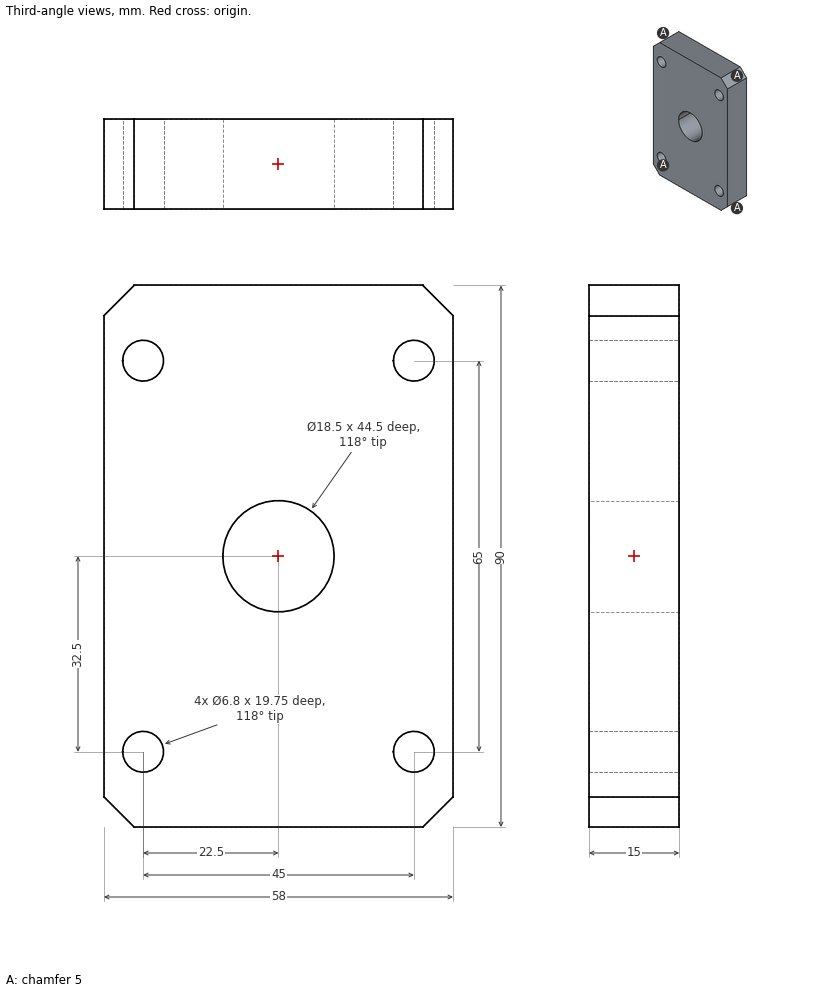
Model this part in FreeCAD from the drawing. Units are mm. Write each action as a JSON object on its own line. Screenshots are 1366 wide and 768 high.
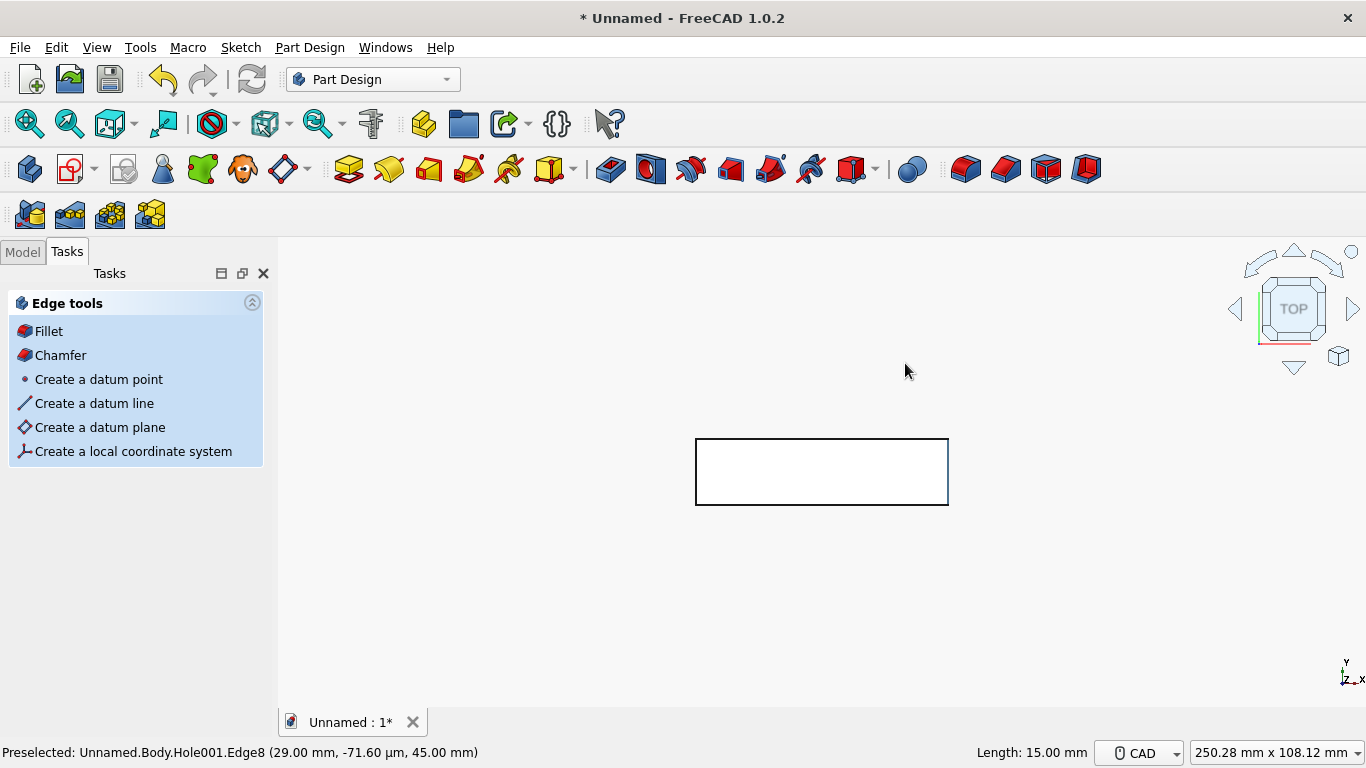
{"action": "left_click", "coordinate": [30, 124]}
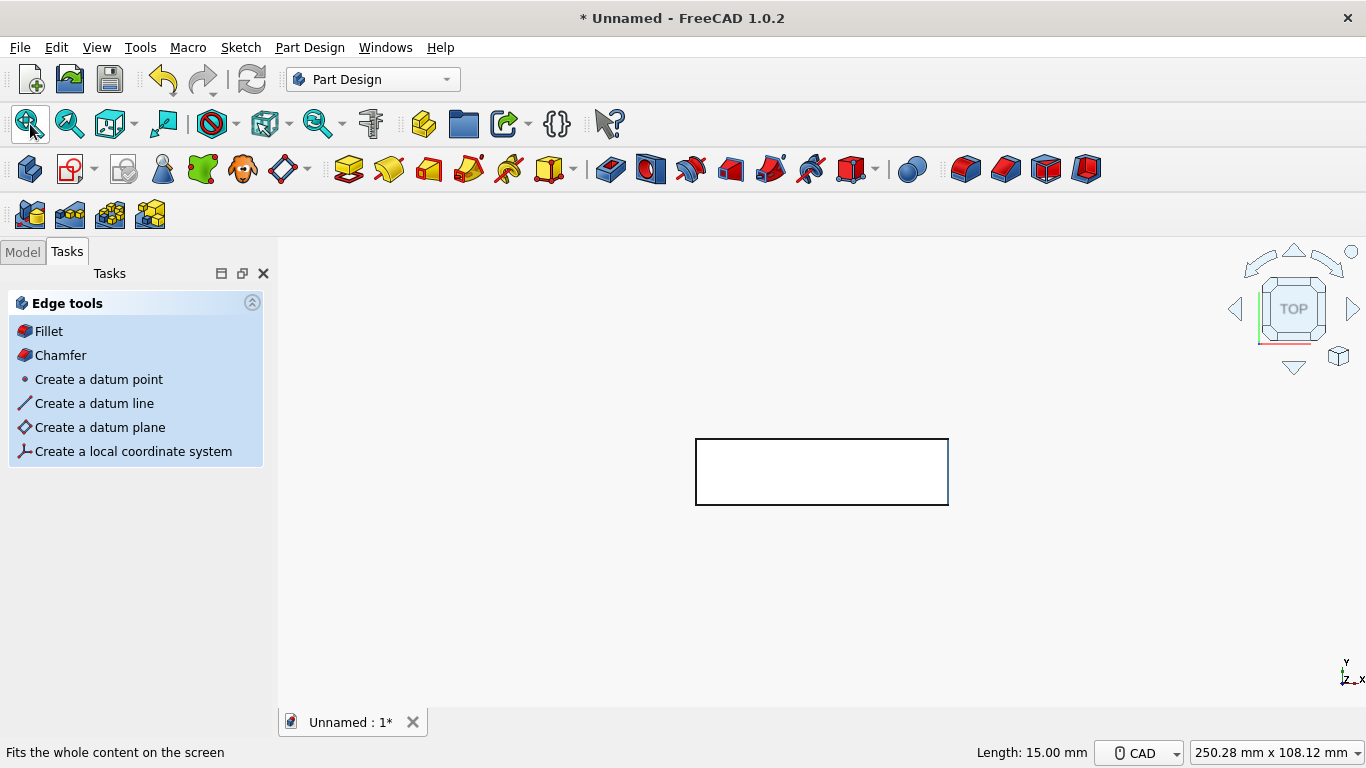
{"action": "left_click", "coordinate": [696, 471], "text": "ctrl"}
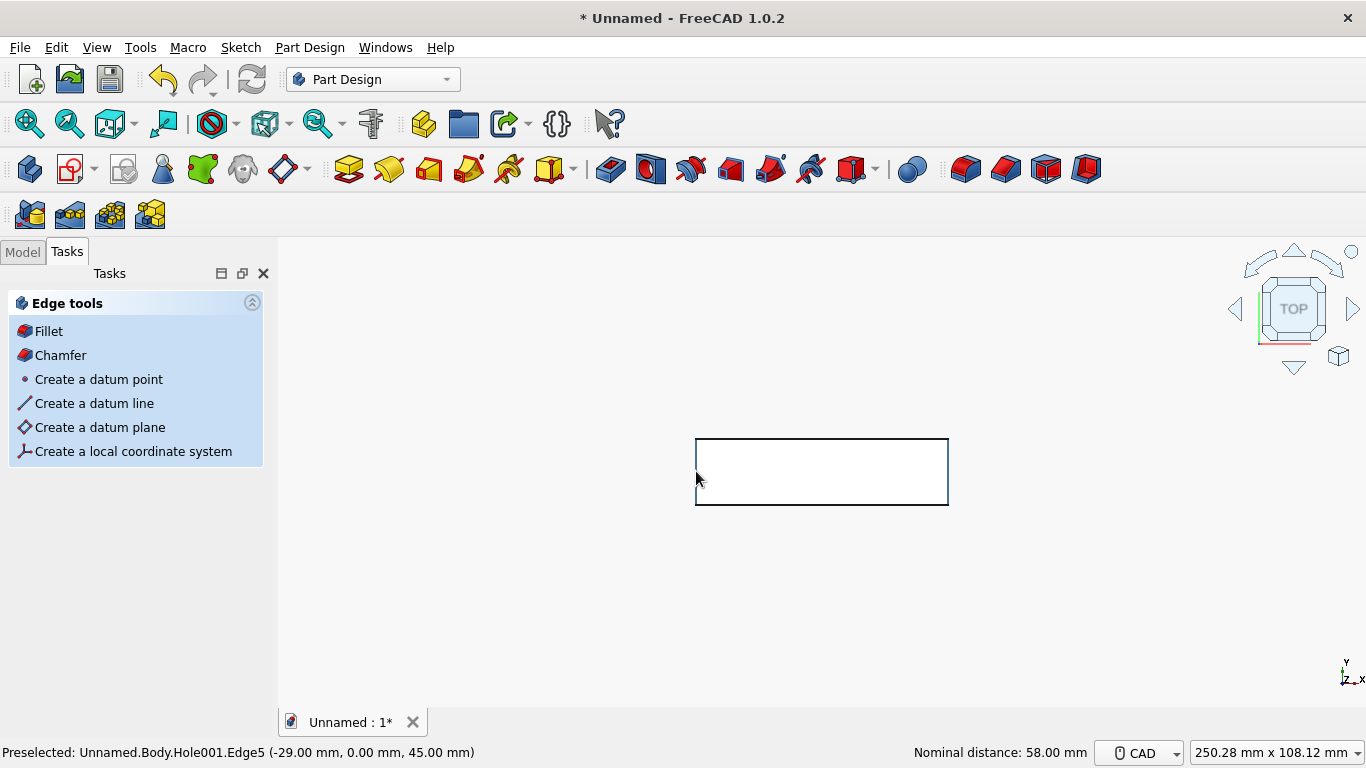
{"action": "key", "text": "1"}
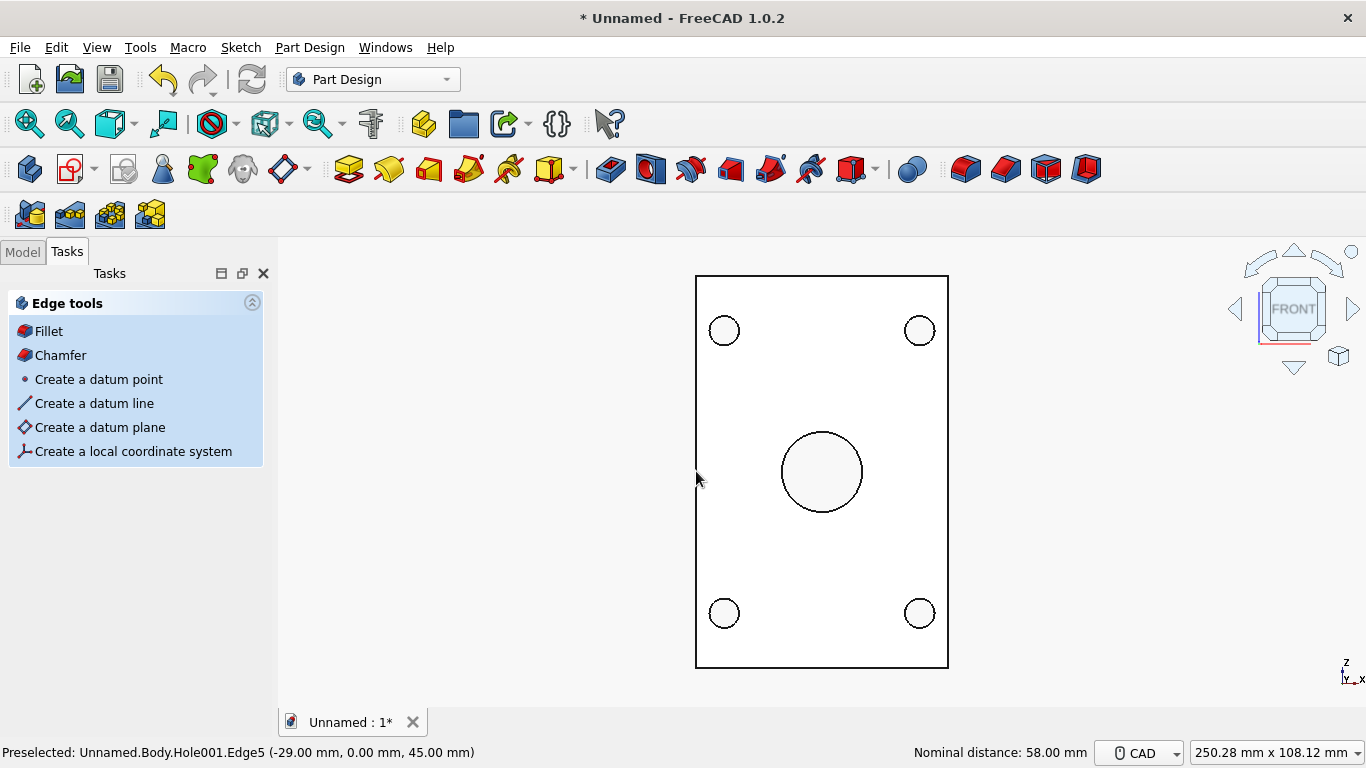
{"action": "key", "text": "3"}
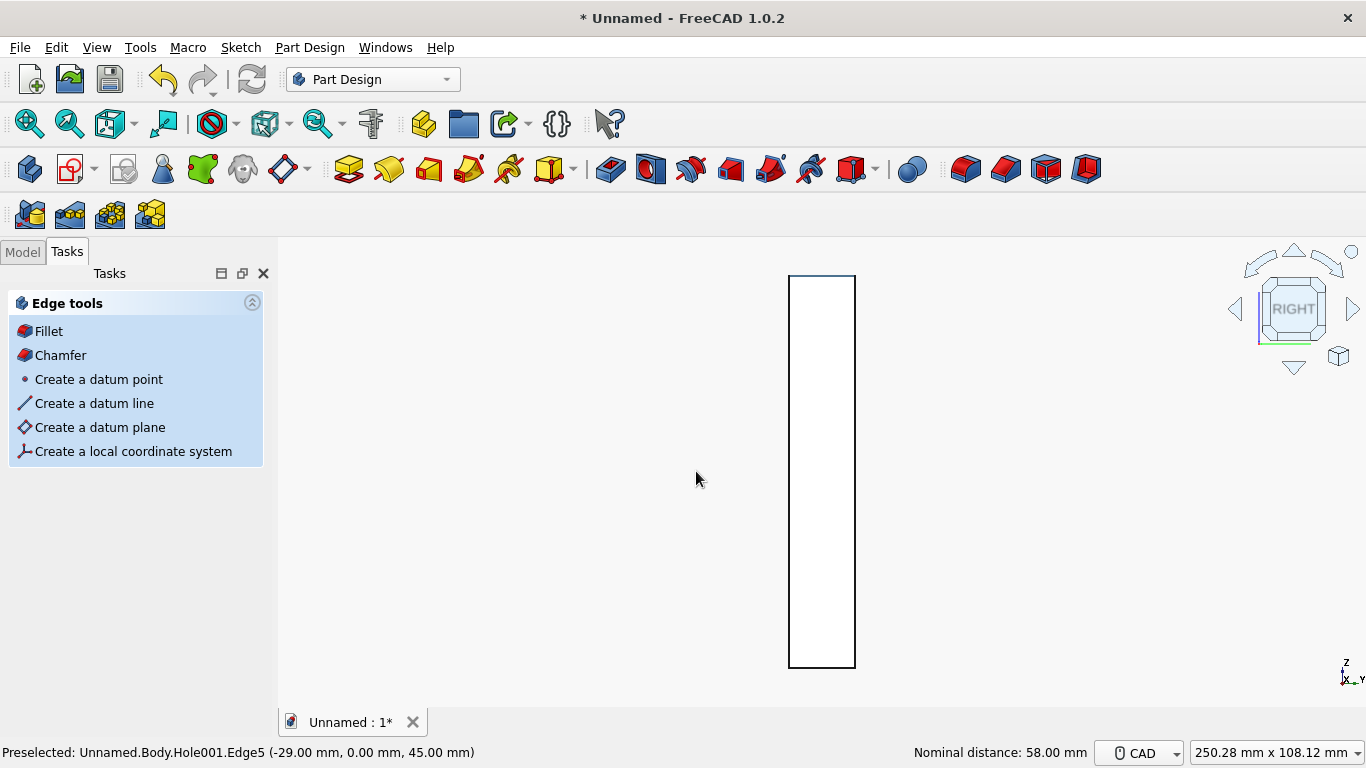
{"action": "left_click", "coordinate": [822, 667], "text": "ctrl"}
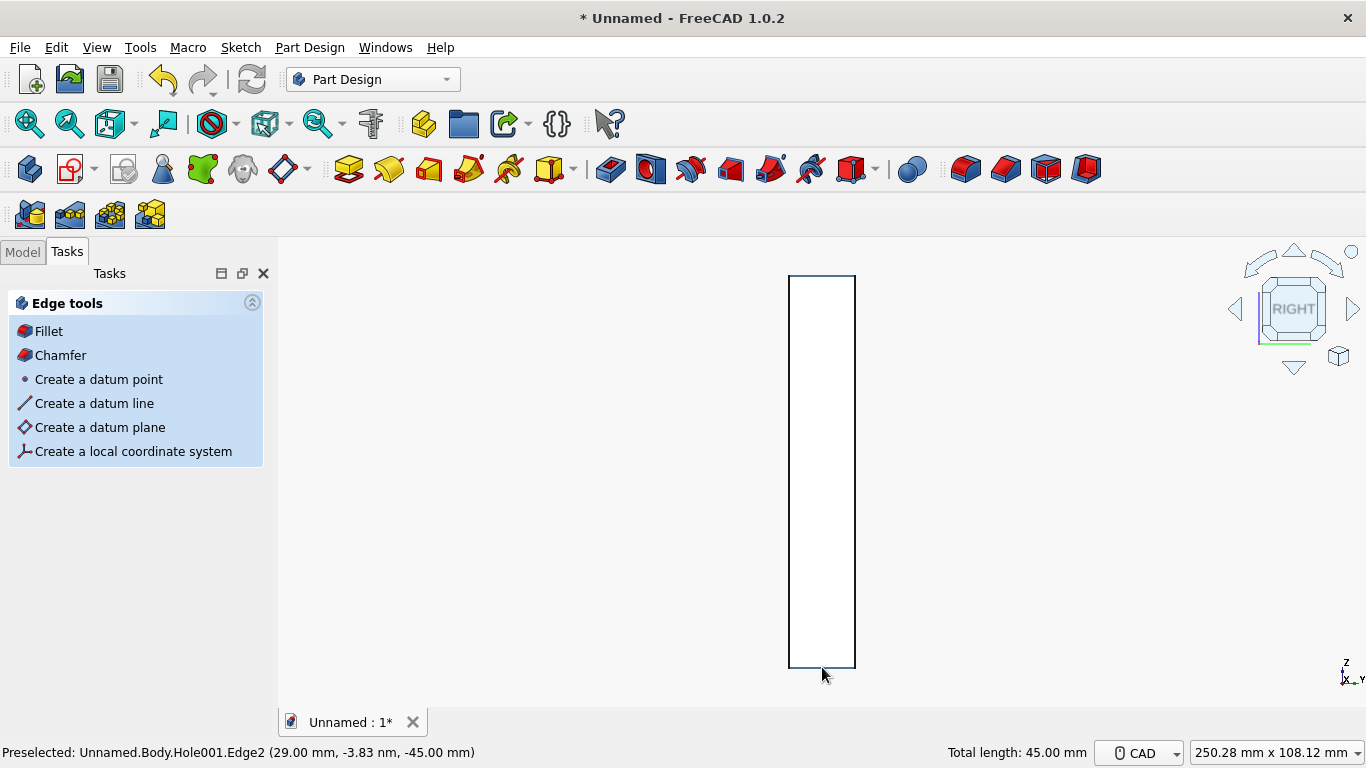
{"action": "key", "text": "5"}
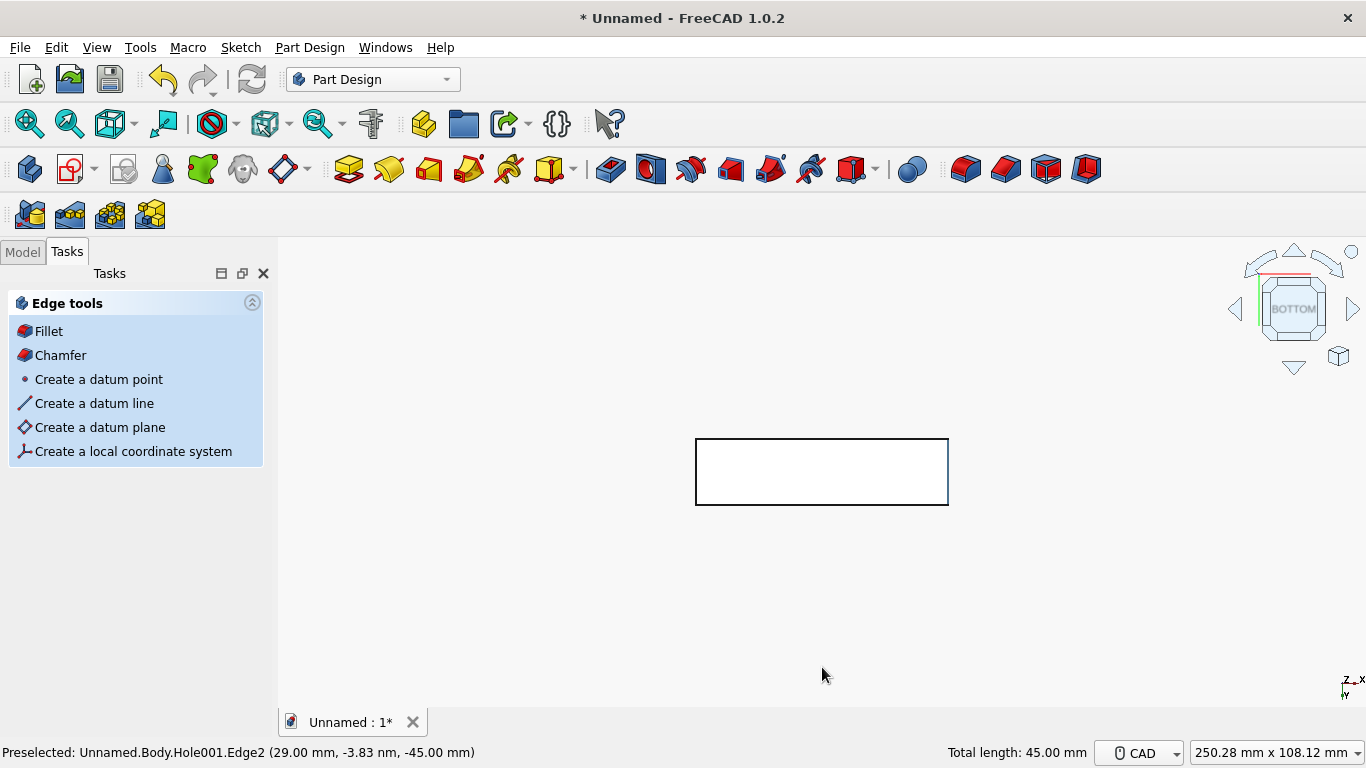
{"action": "left_click", "coordinate": [30, 124]}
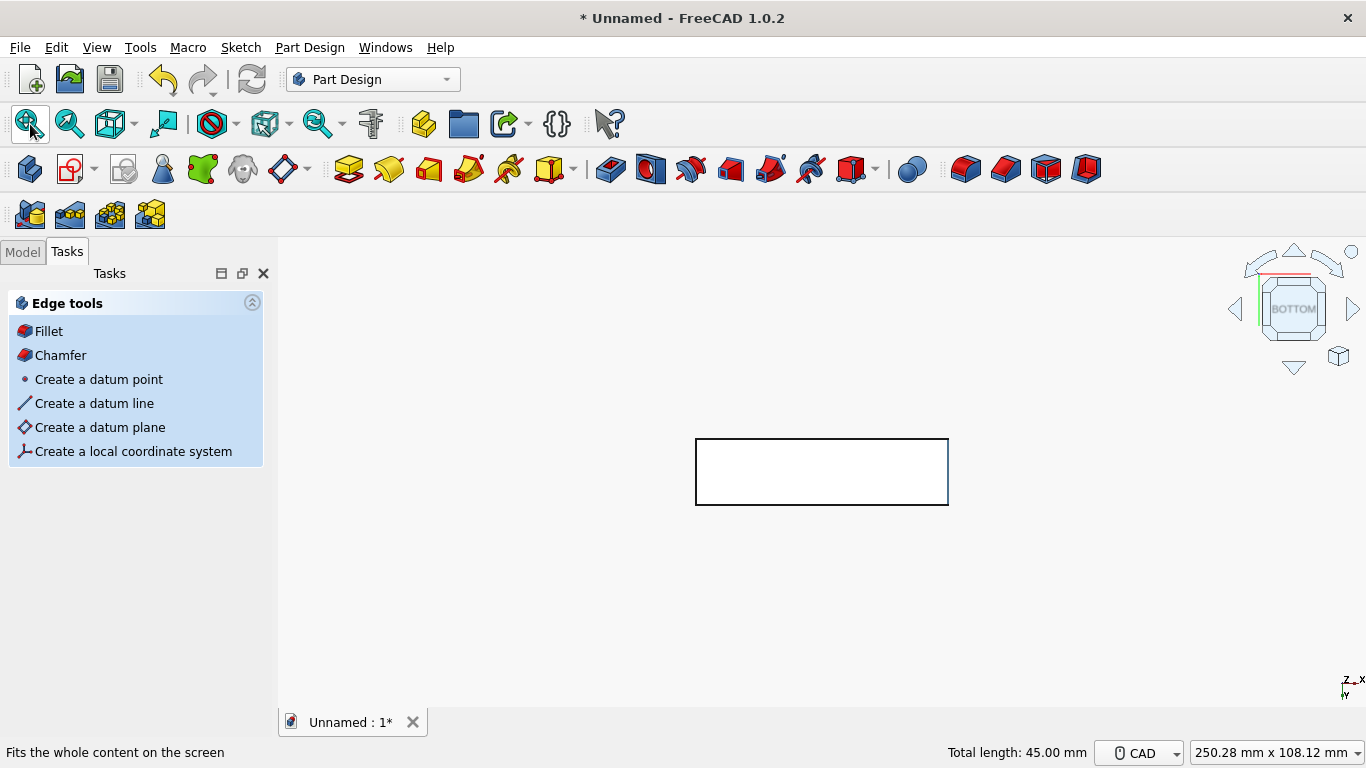
{"action": "left_click", "coordinate": [696, 471], "text": "ctrl"}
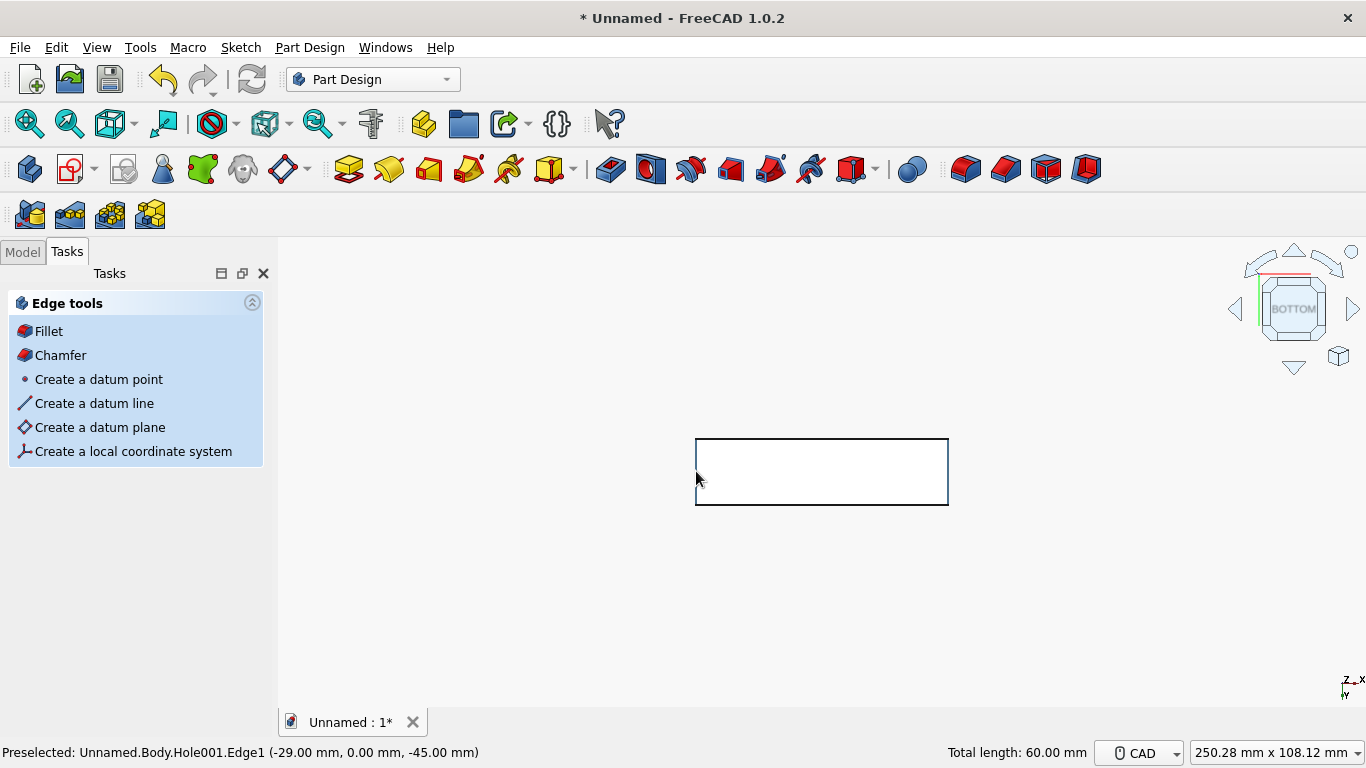
{"action": "left_click", "coordinate": [1006, 170]}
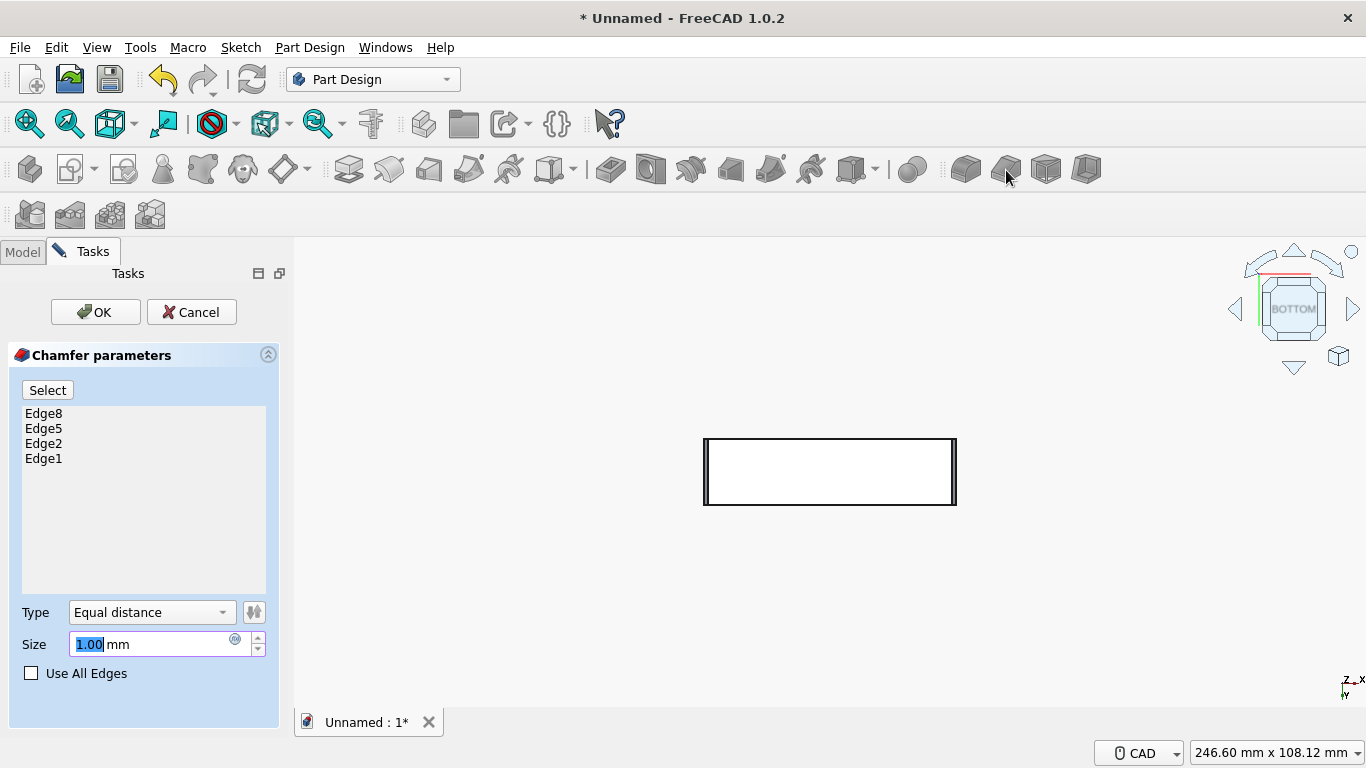
{"action": "type", "text": "5"}
{"action": "key", "text": "Tab"}